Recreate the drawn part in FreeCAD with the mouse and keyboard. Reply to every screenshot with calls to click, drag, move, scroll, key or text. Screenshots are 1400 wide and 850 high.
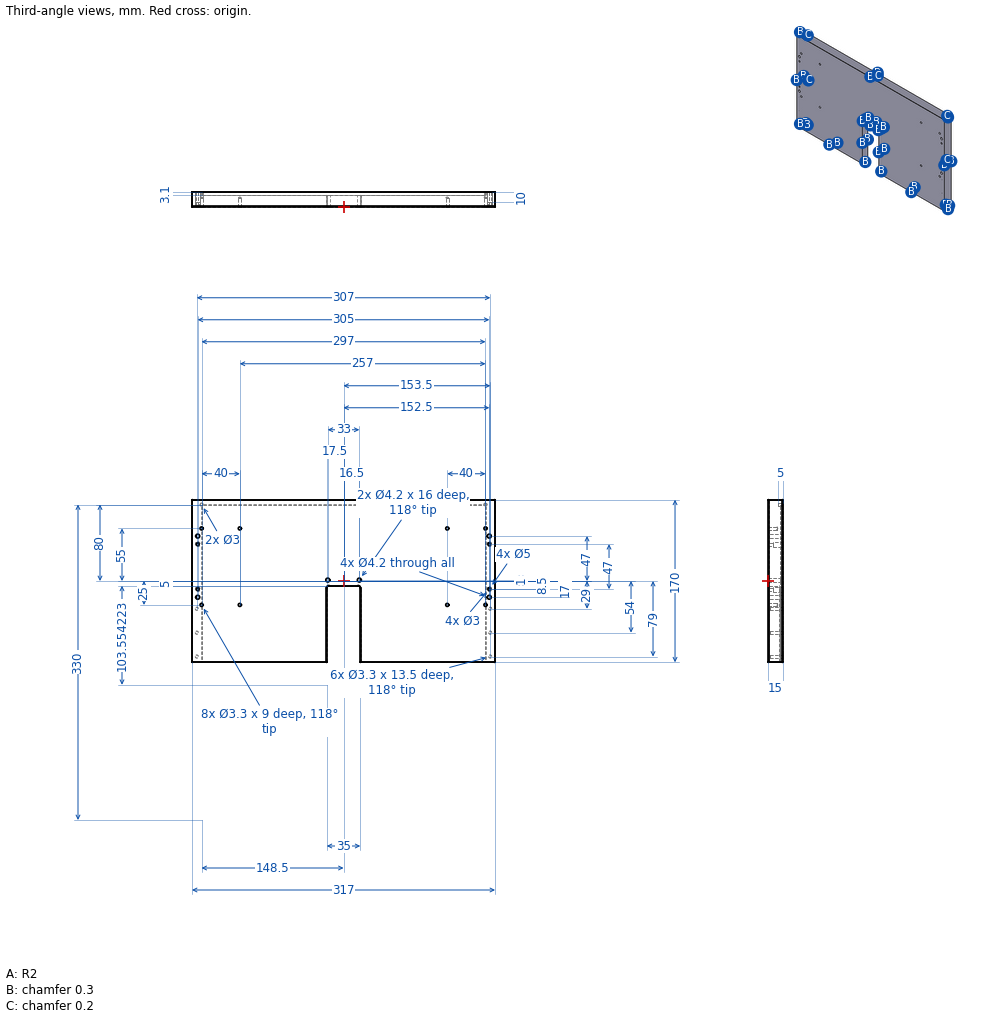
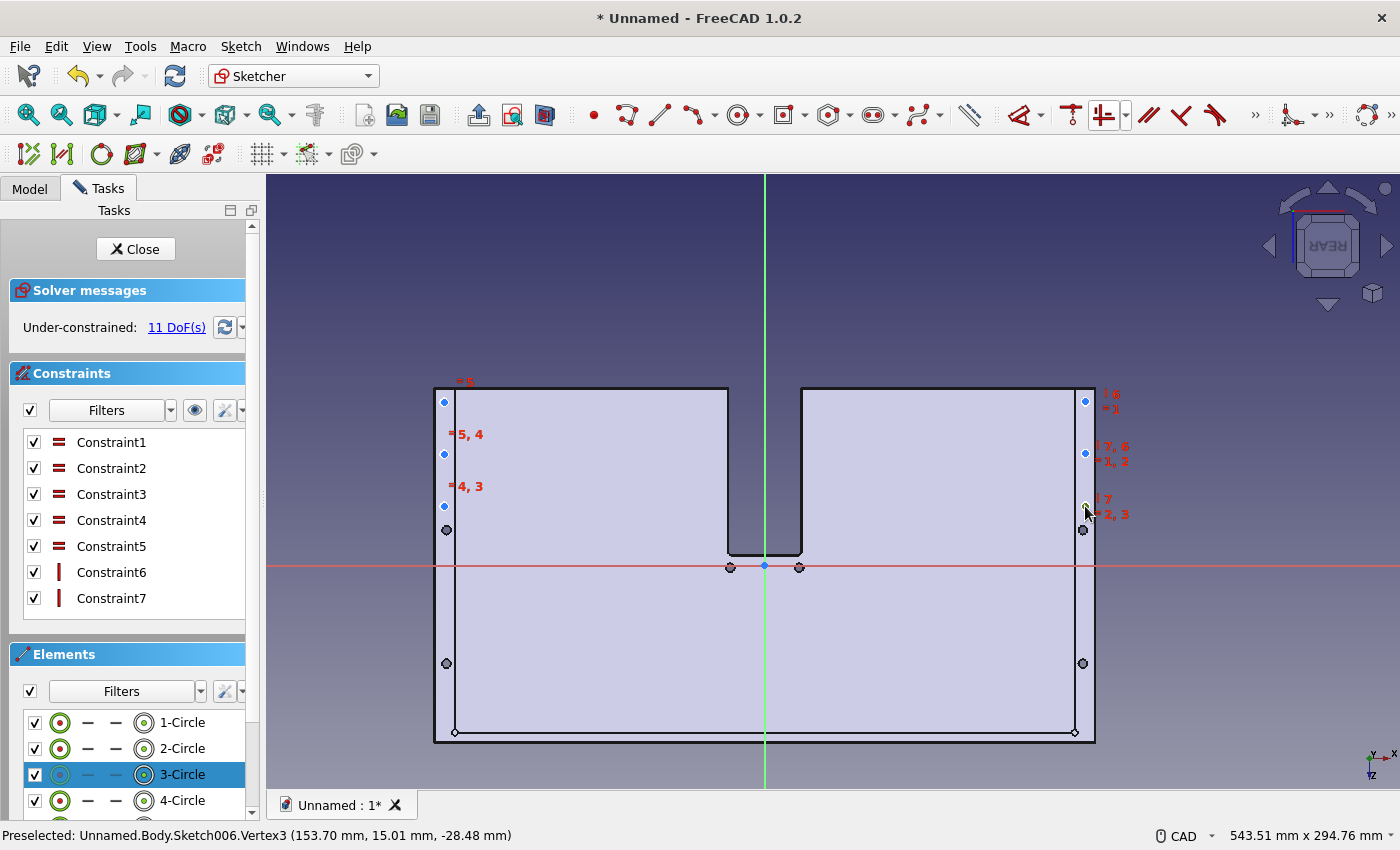
click(444, 506)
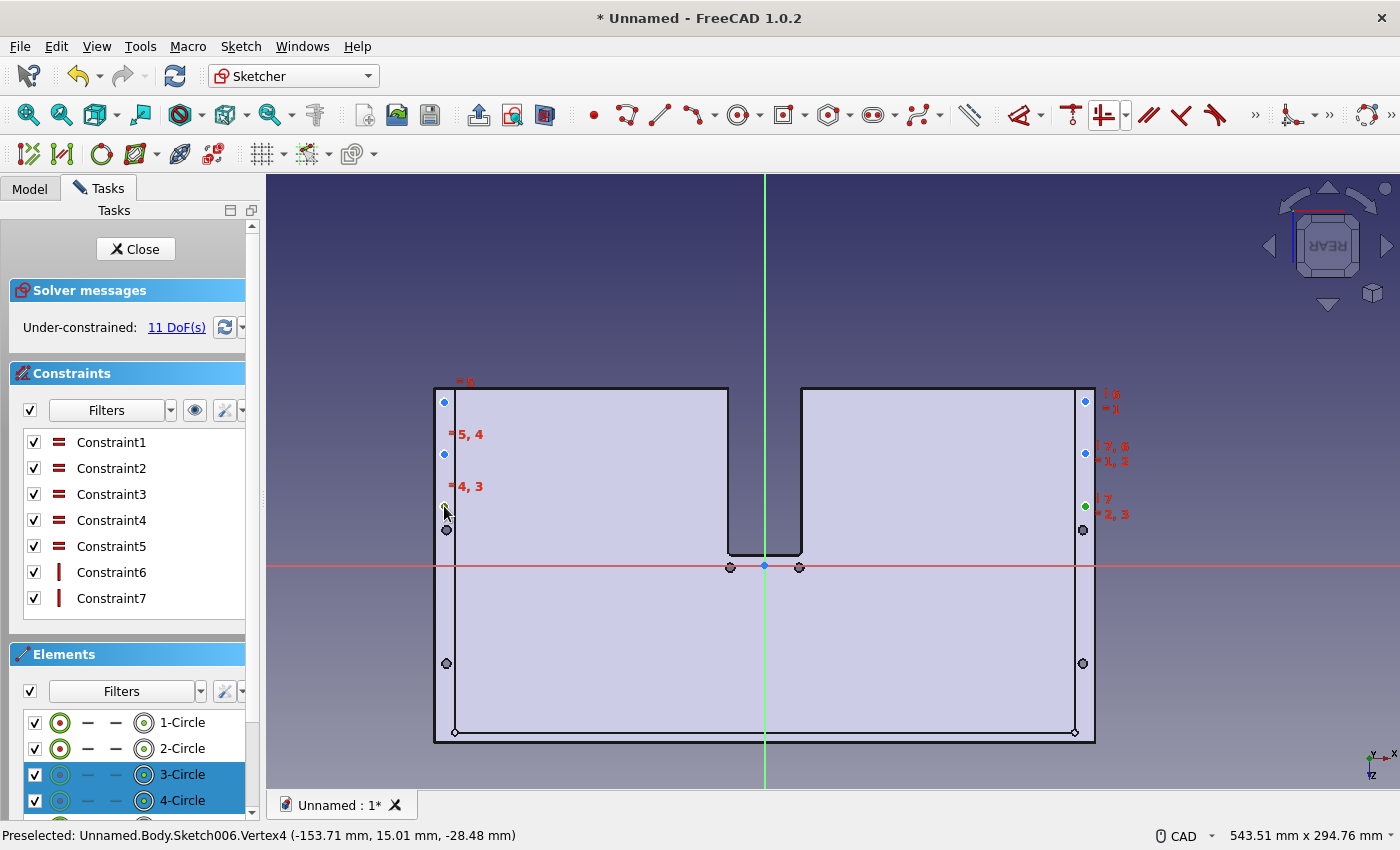
key(h)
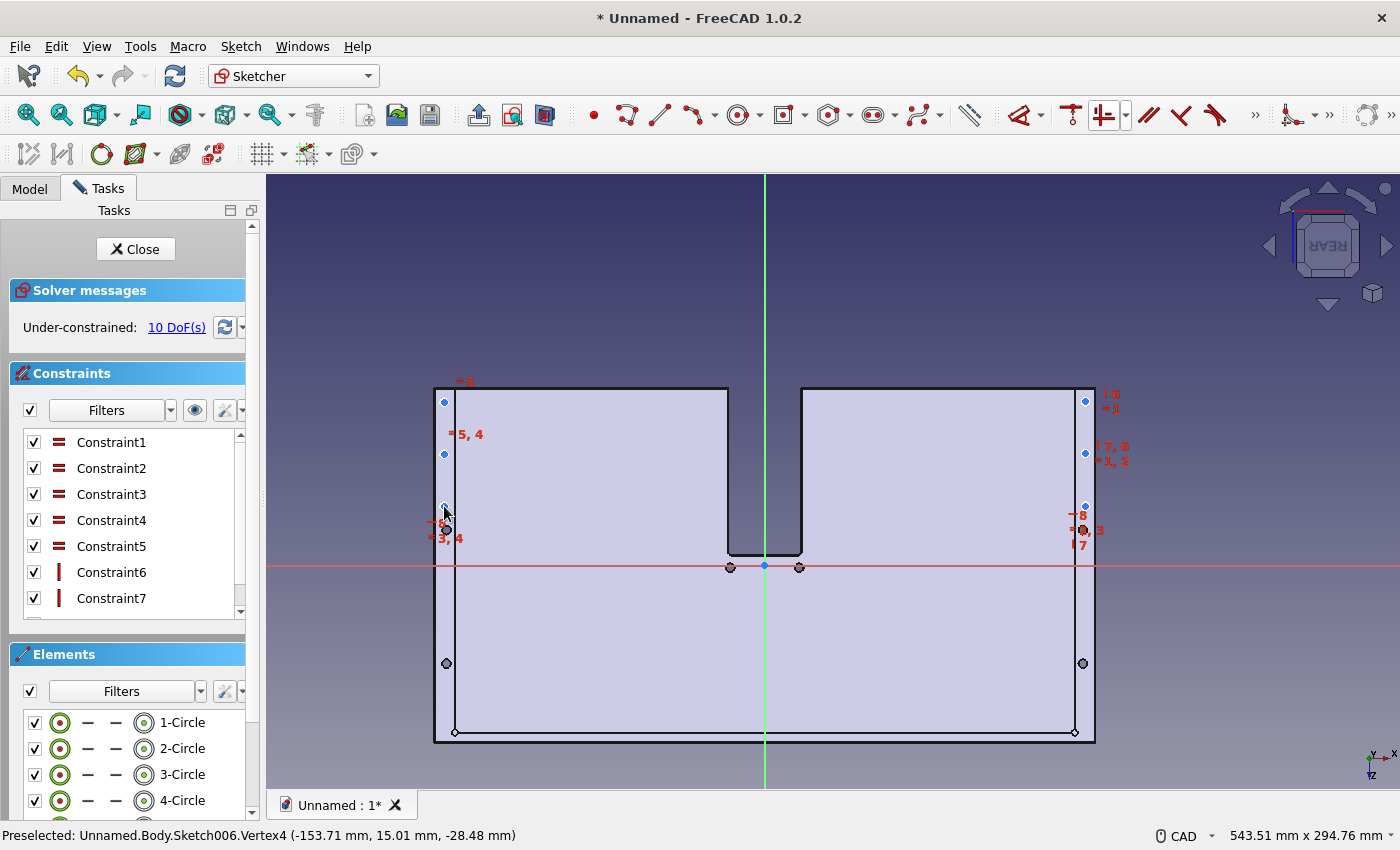
click(444, 506)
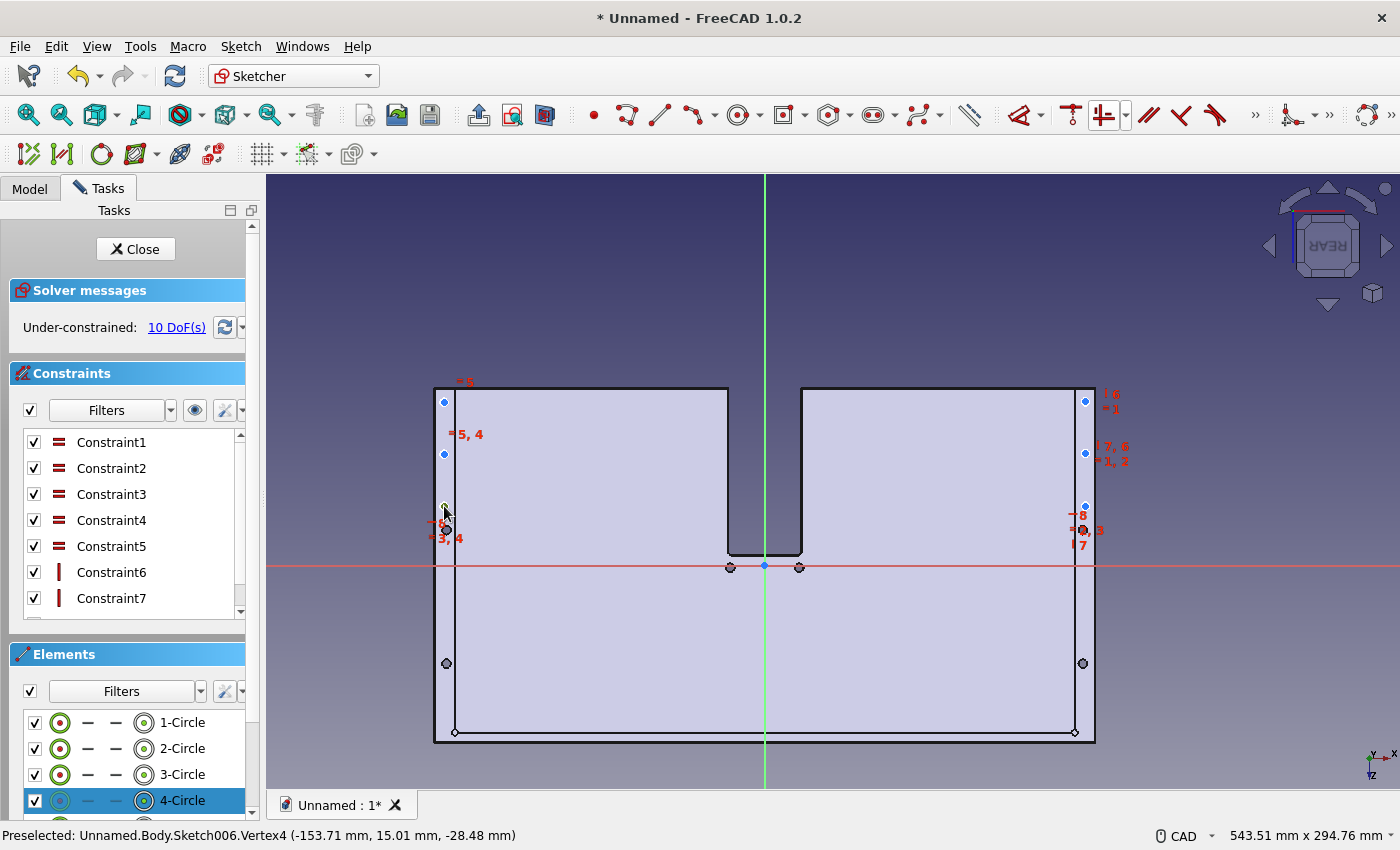
click(444, 454)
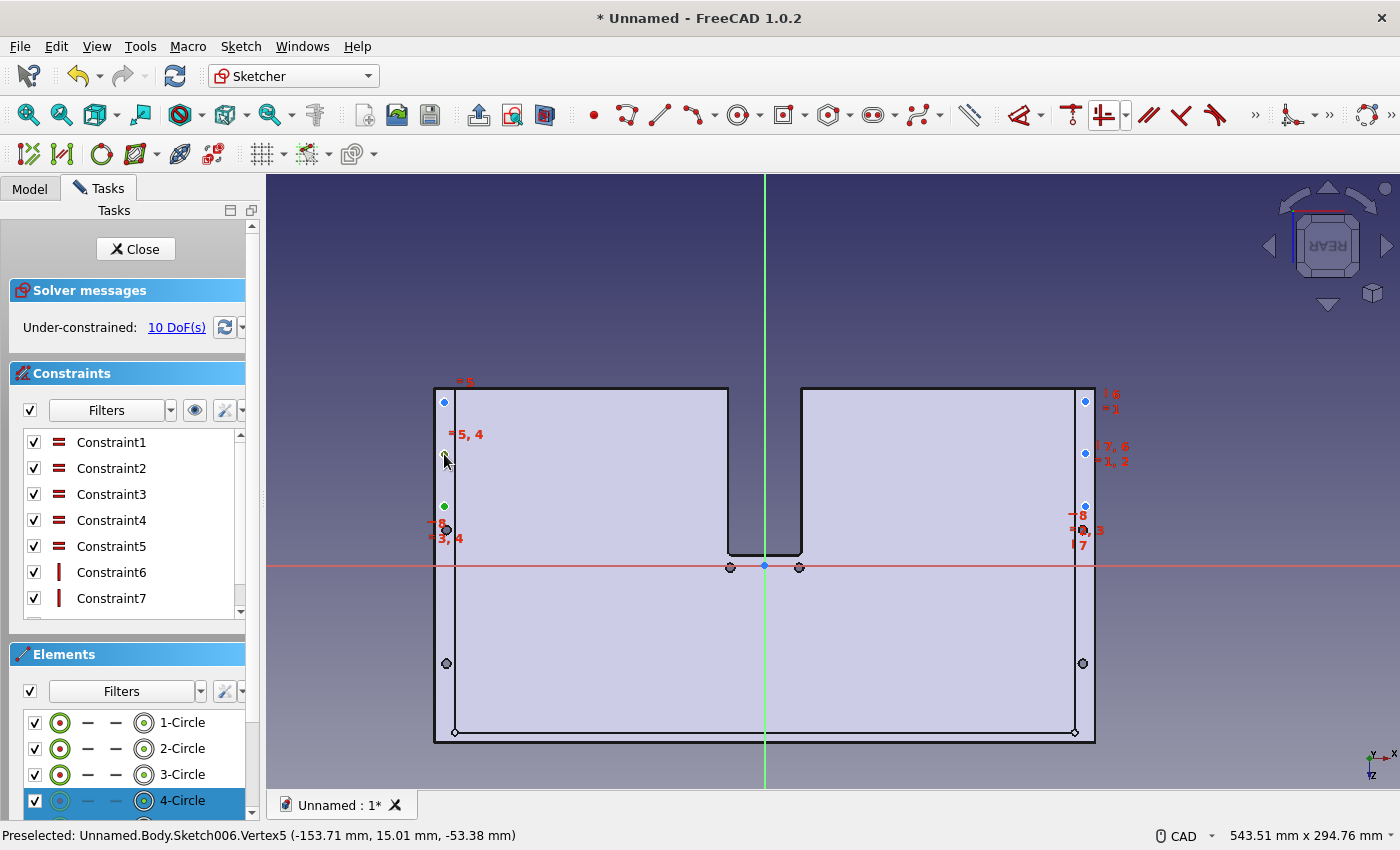
key(v)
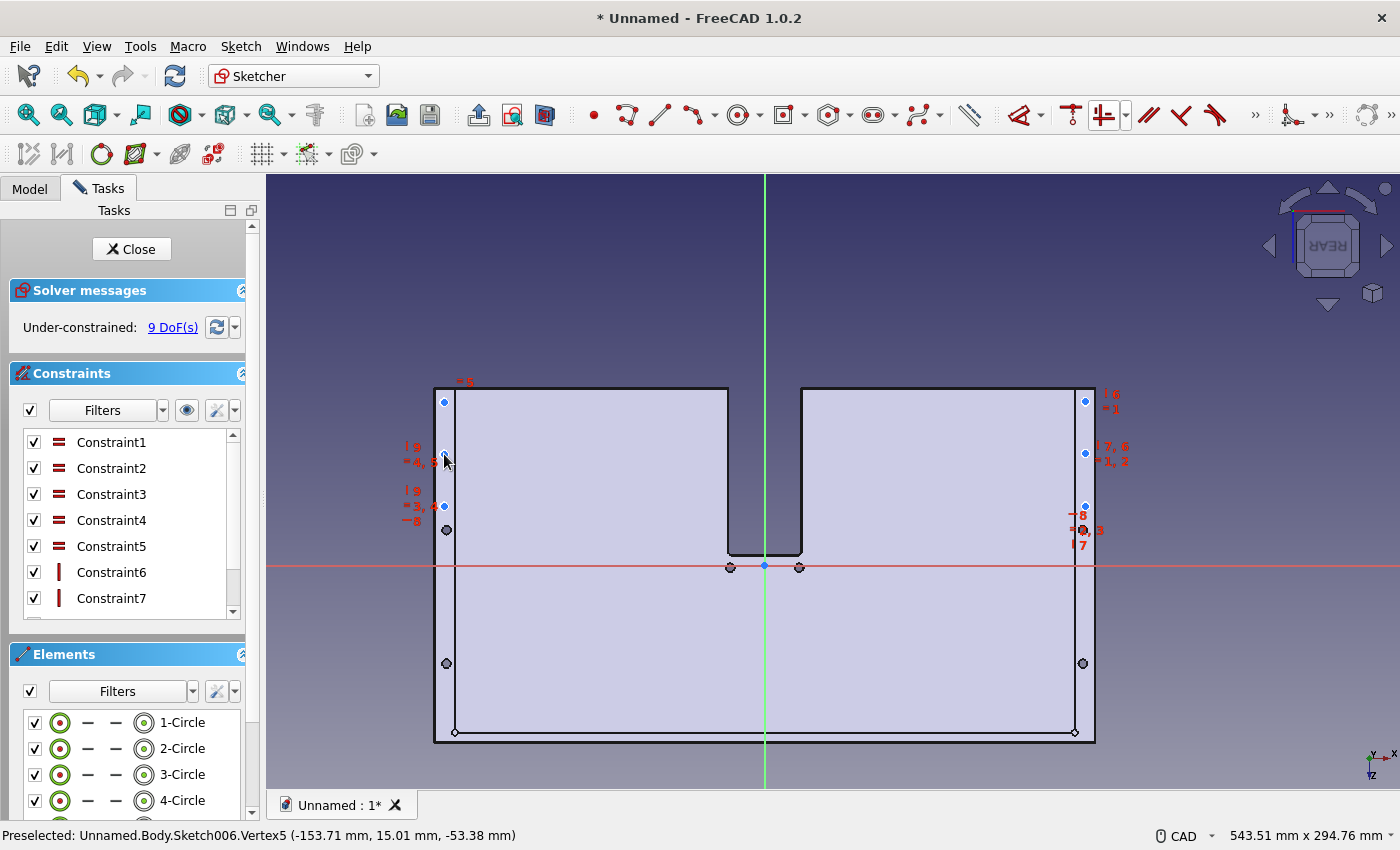
click(1085, 453)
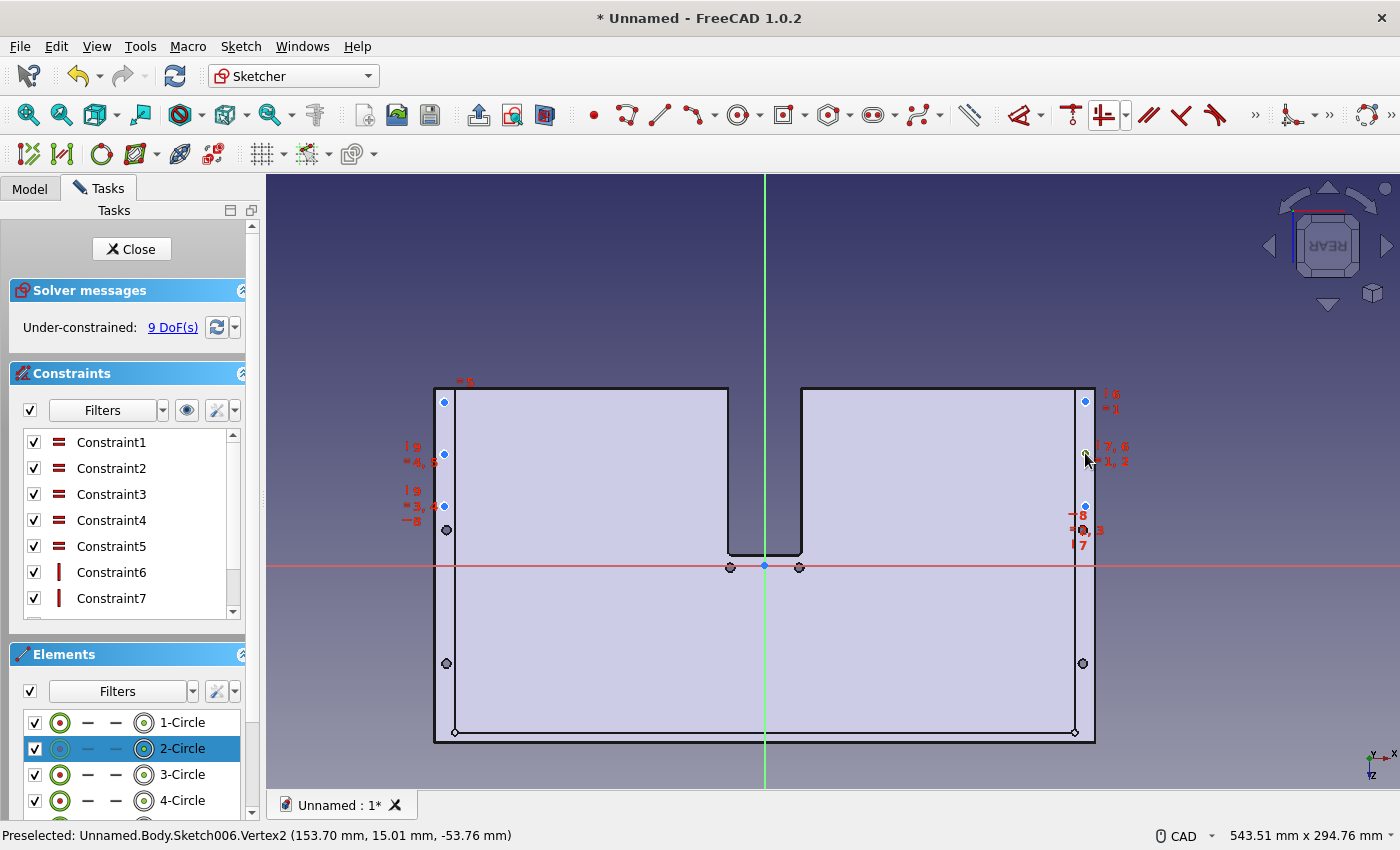
click(444, 454)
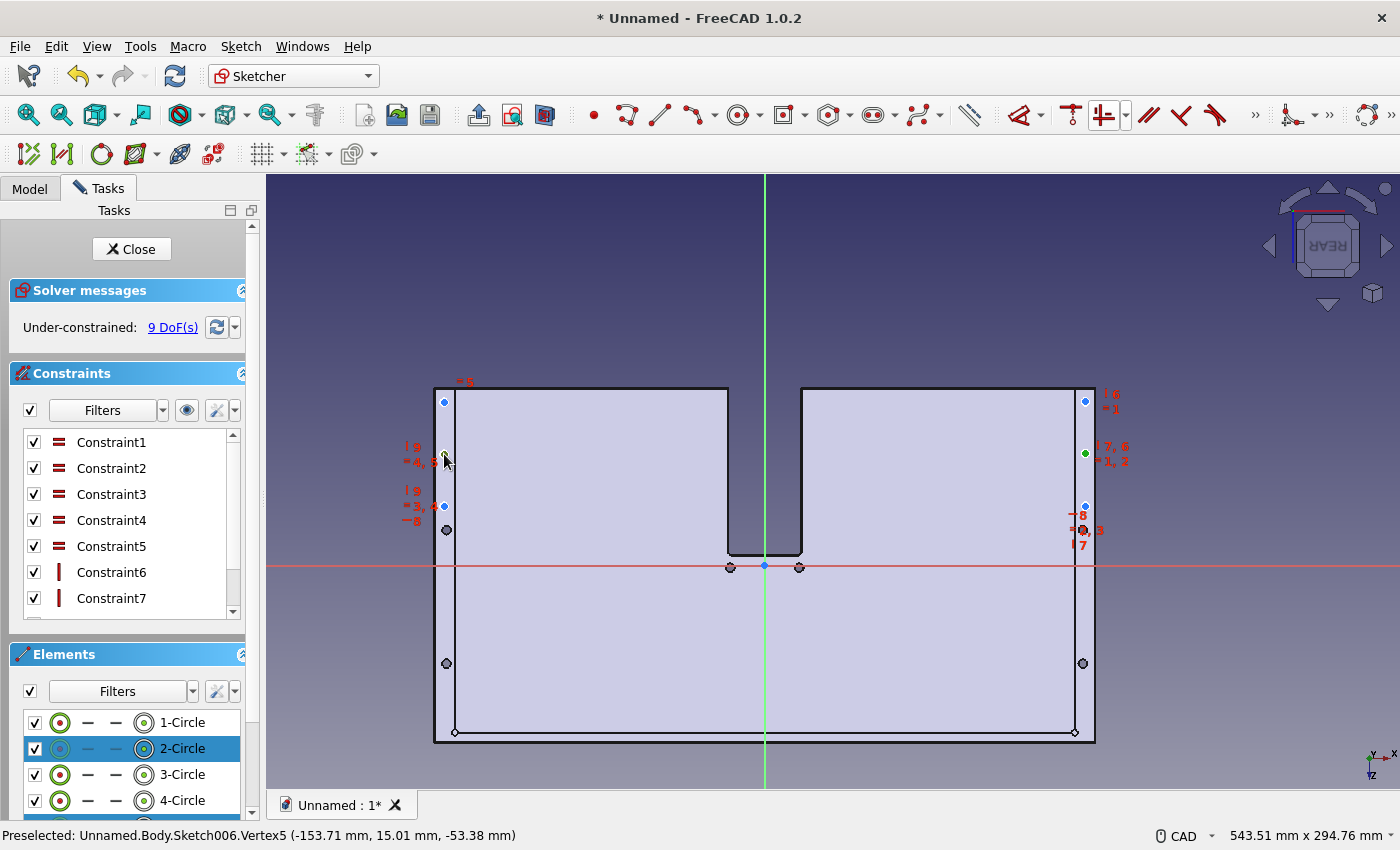
key(h)